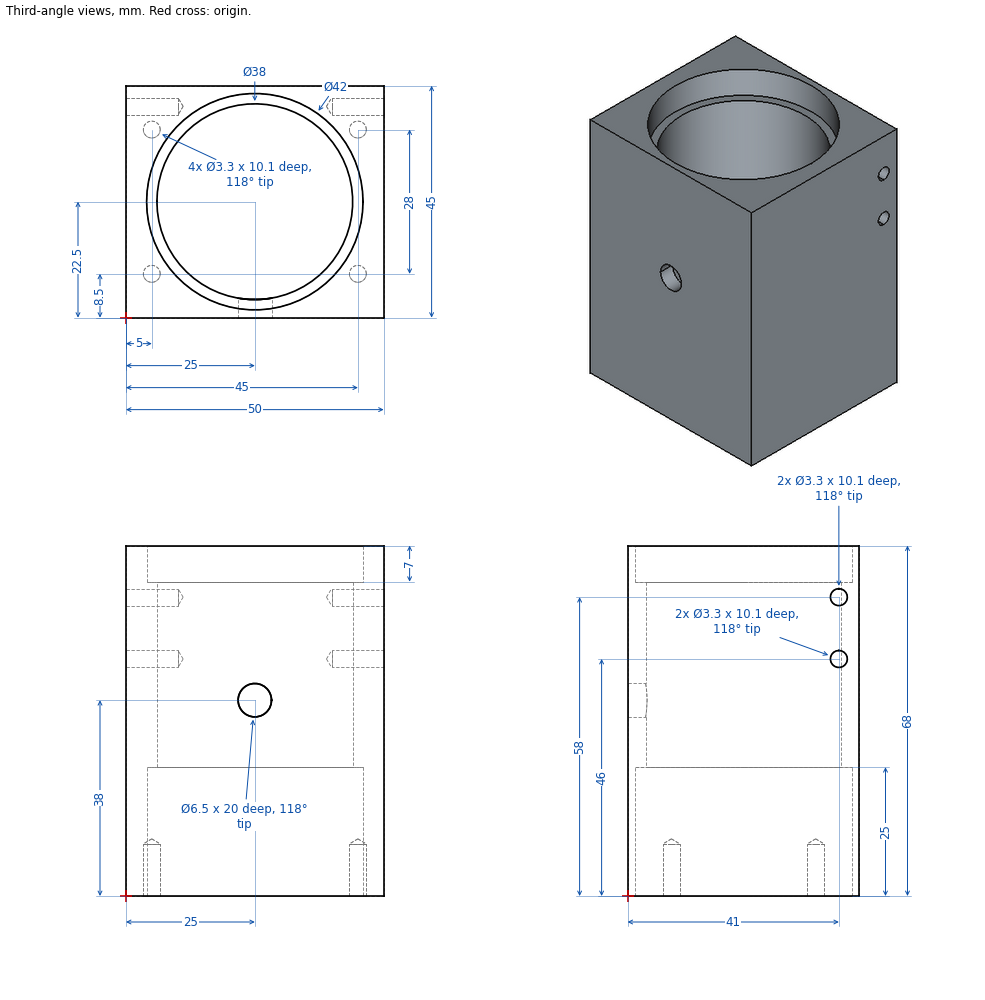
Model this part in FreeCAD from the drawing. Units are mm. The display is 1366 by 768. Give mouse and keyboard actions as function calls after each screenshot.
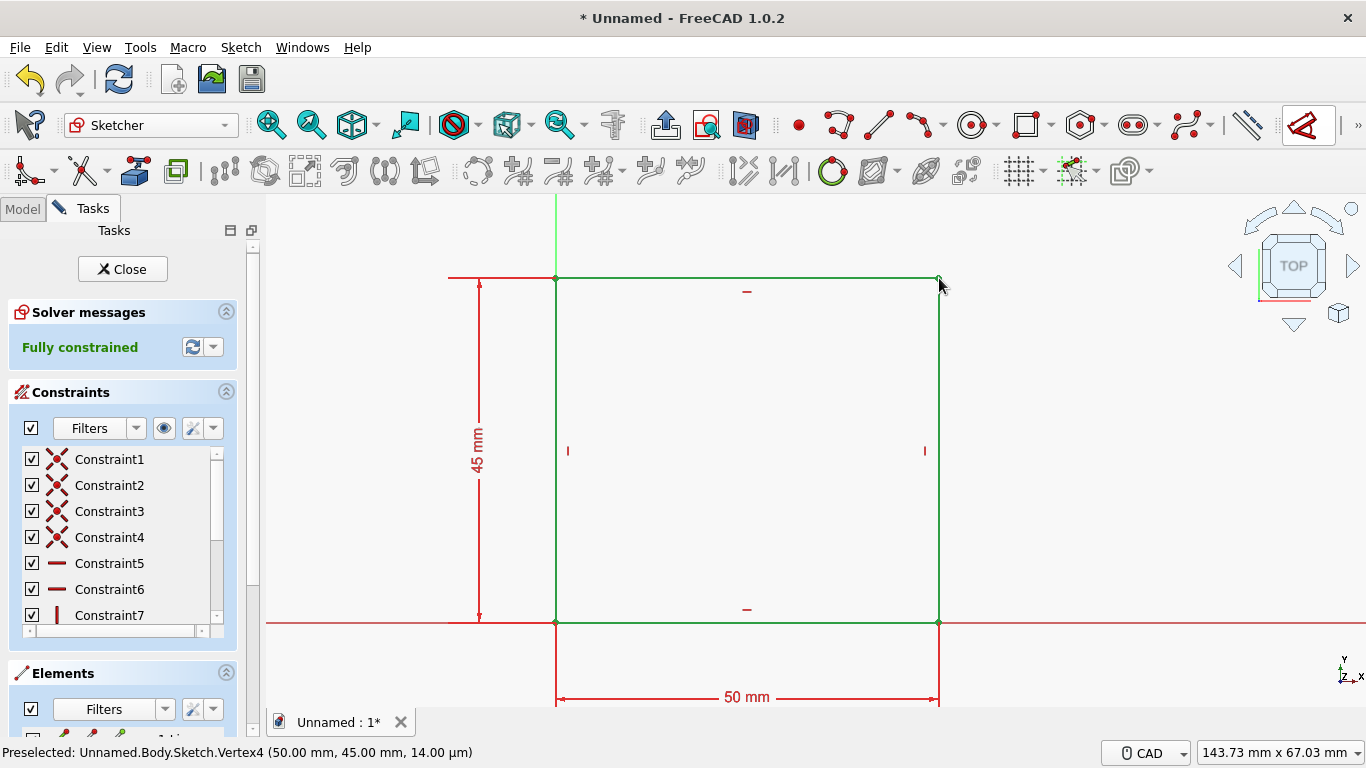
click(123, 269)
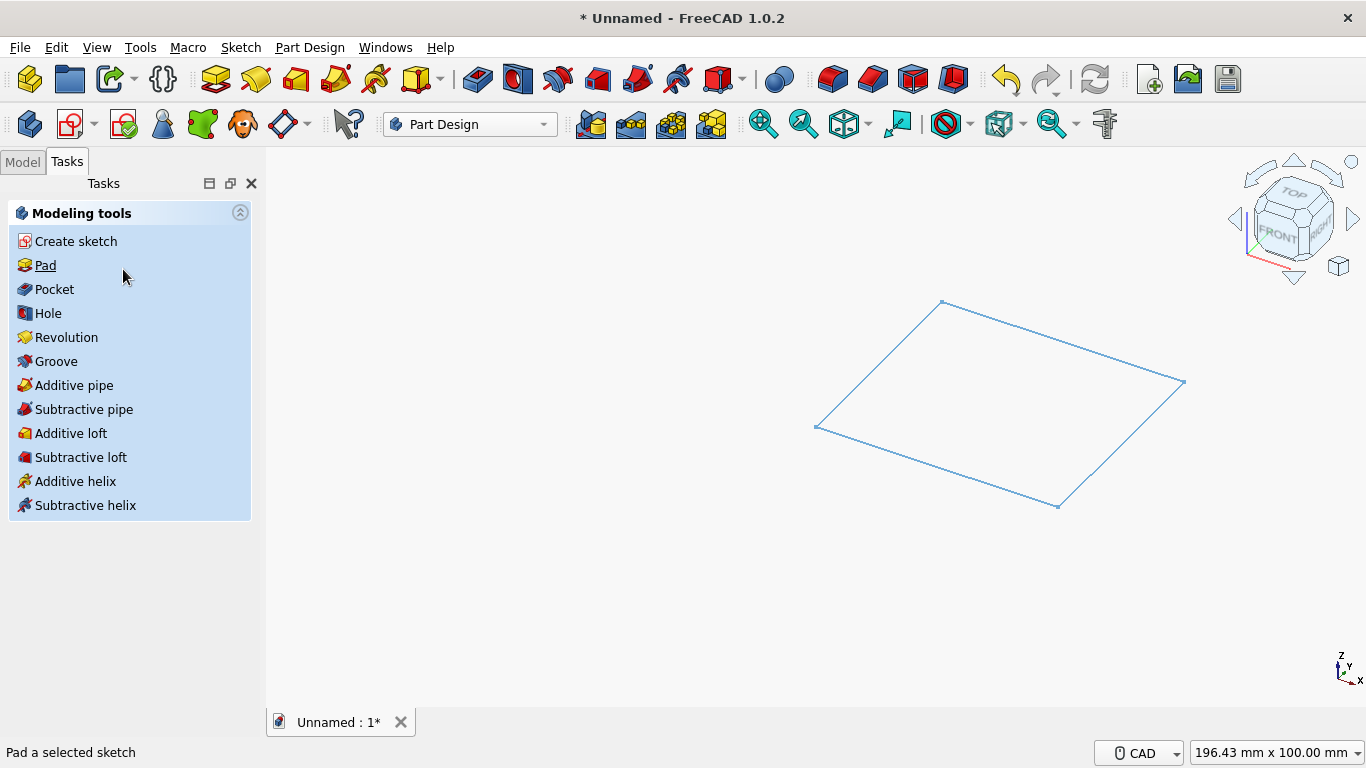
click(216, 80)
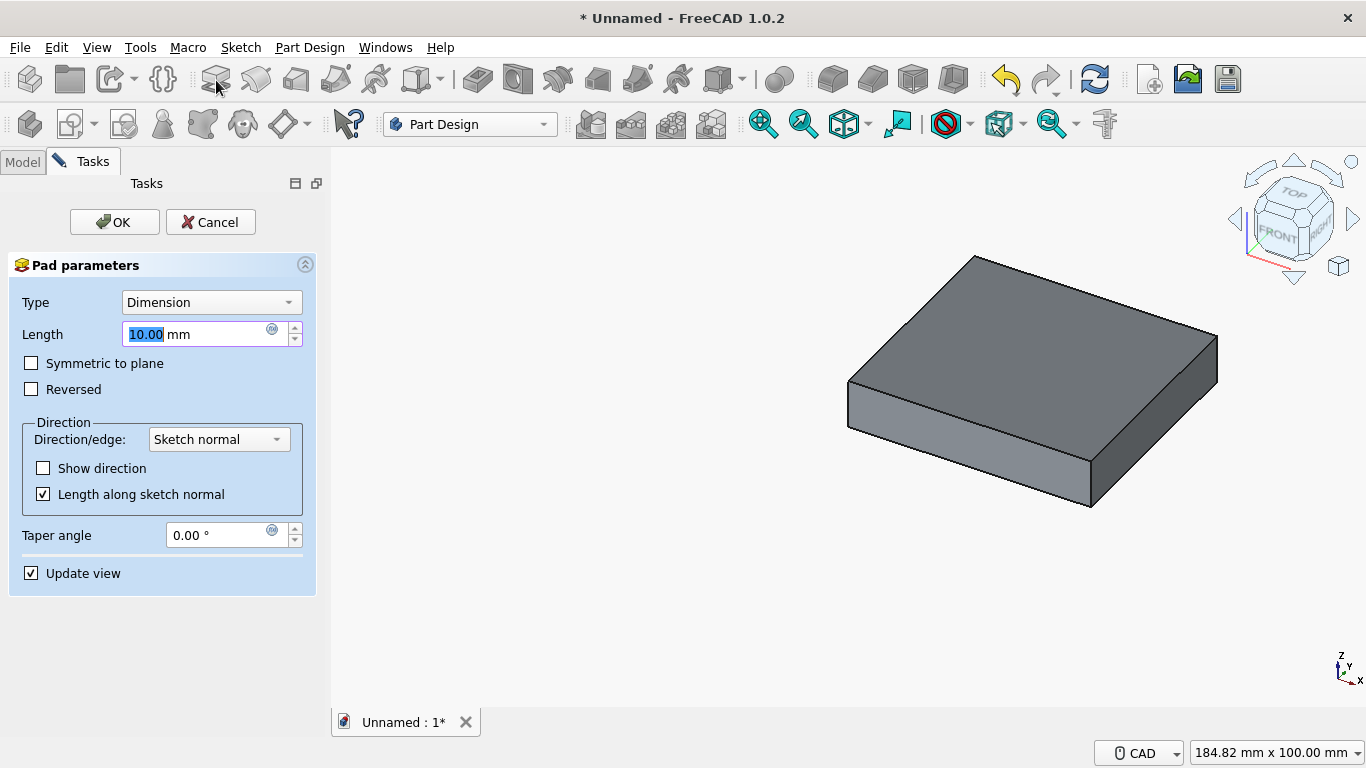
text(68)
key(Tab)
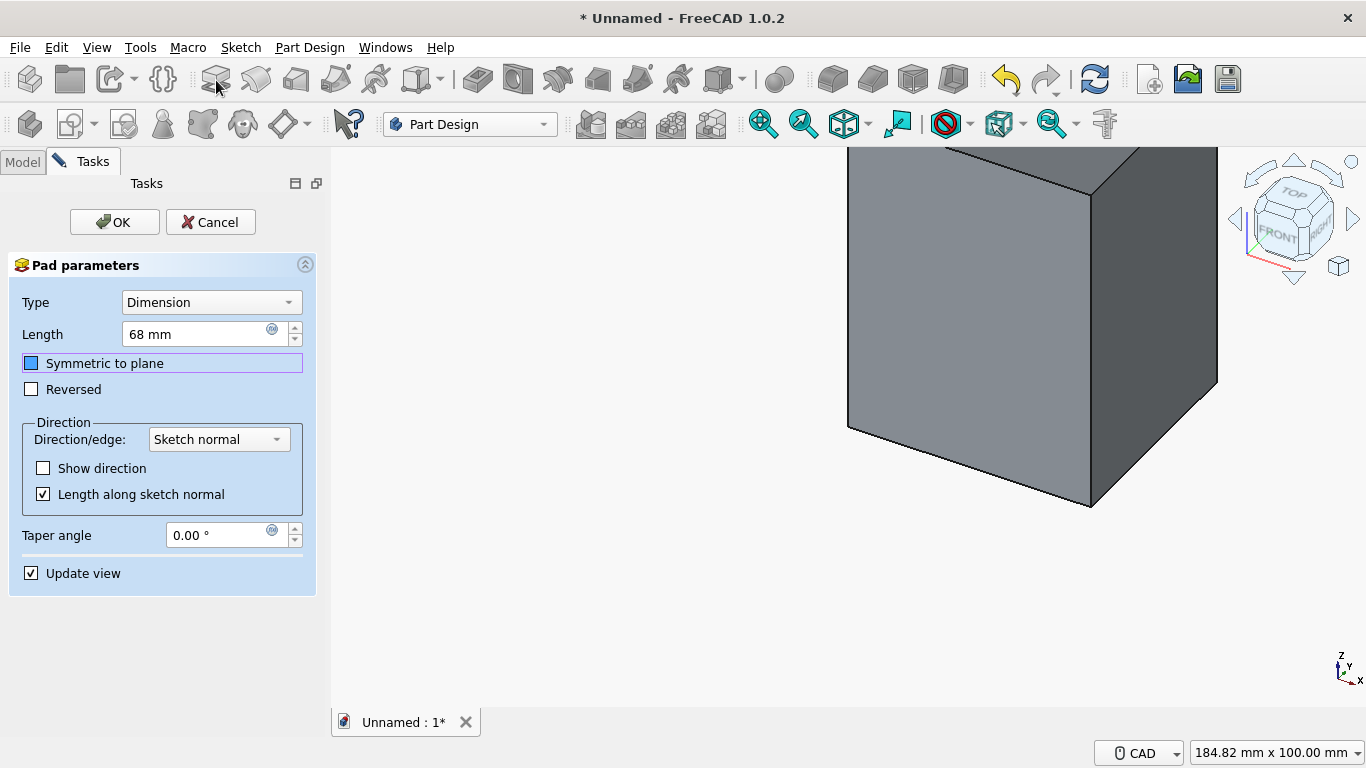
click(115, 222)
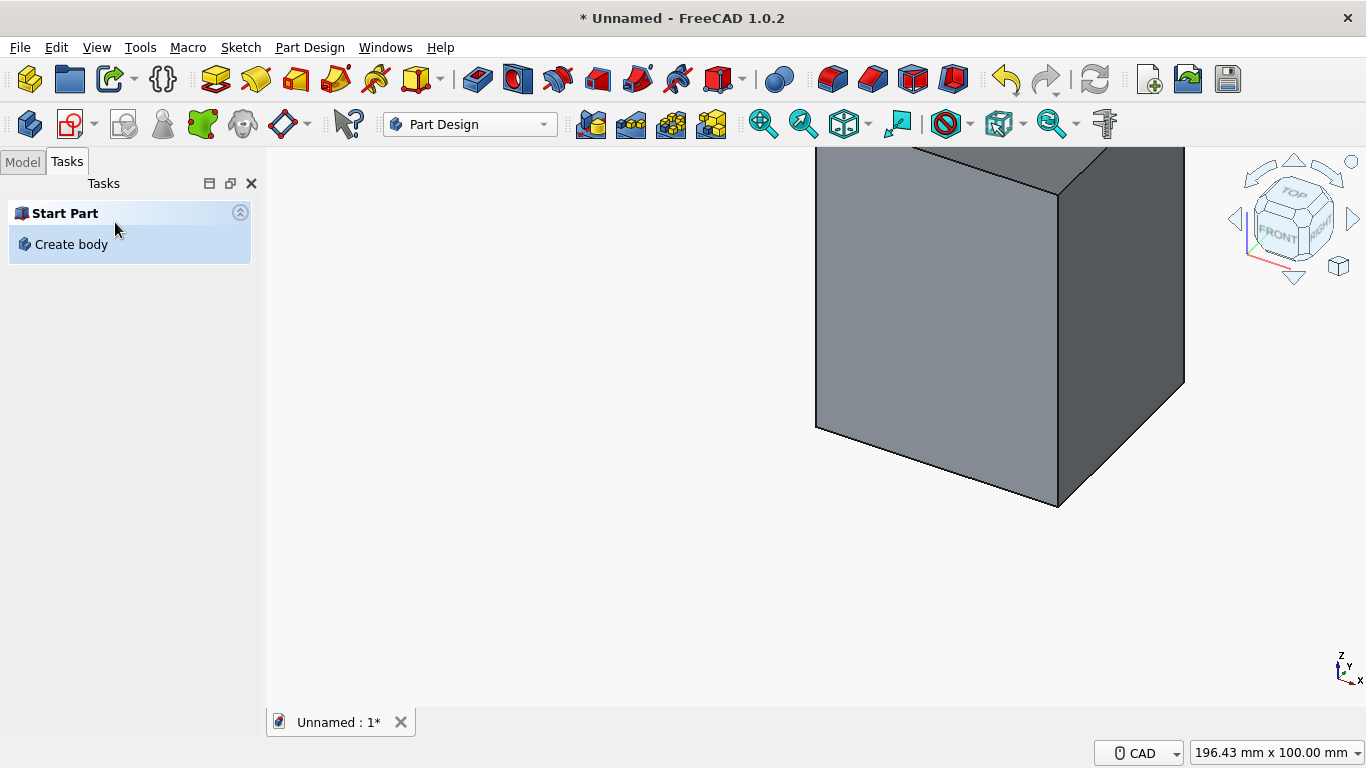
click(764, 124)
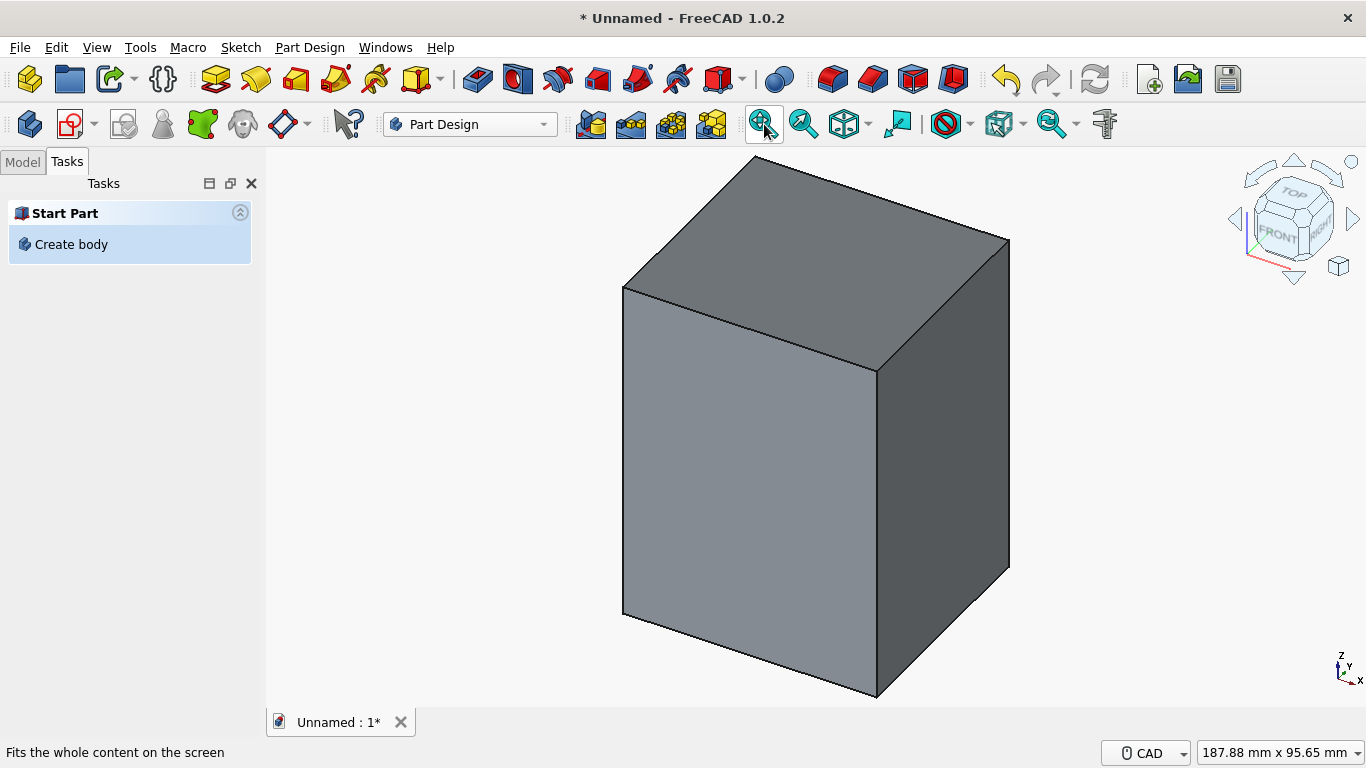
click(70, 124)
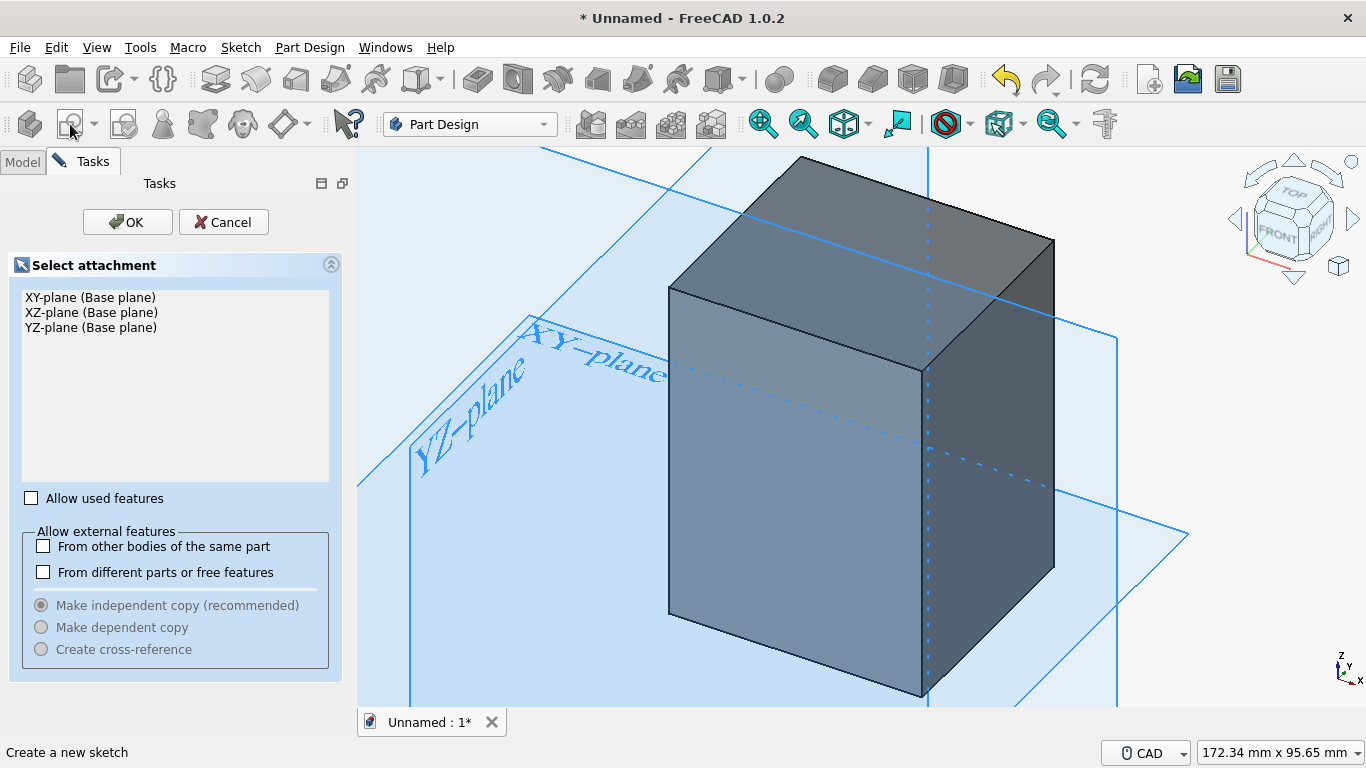
click(82, 298)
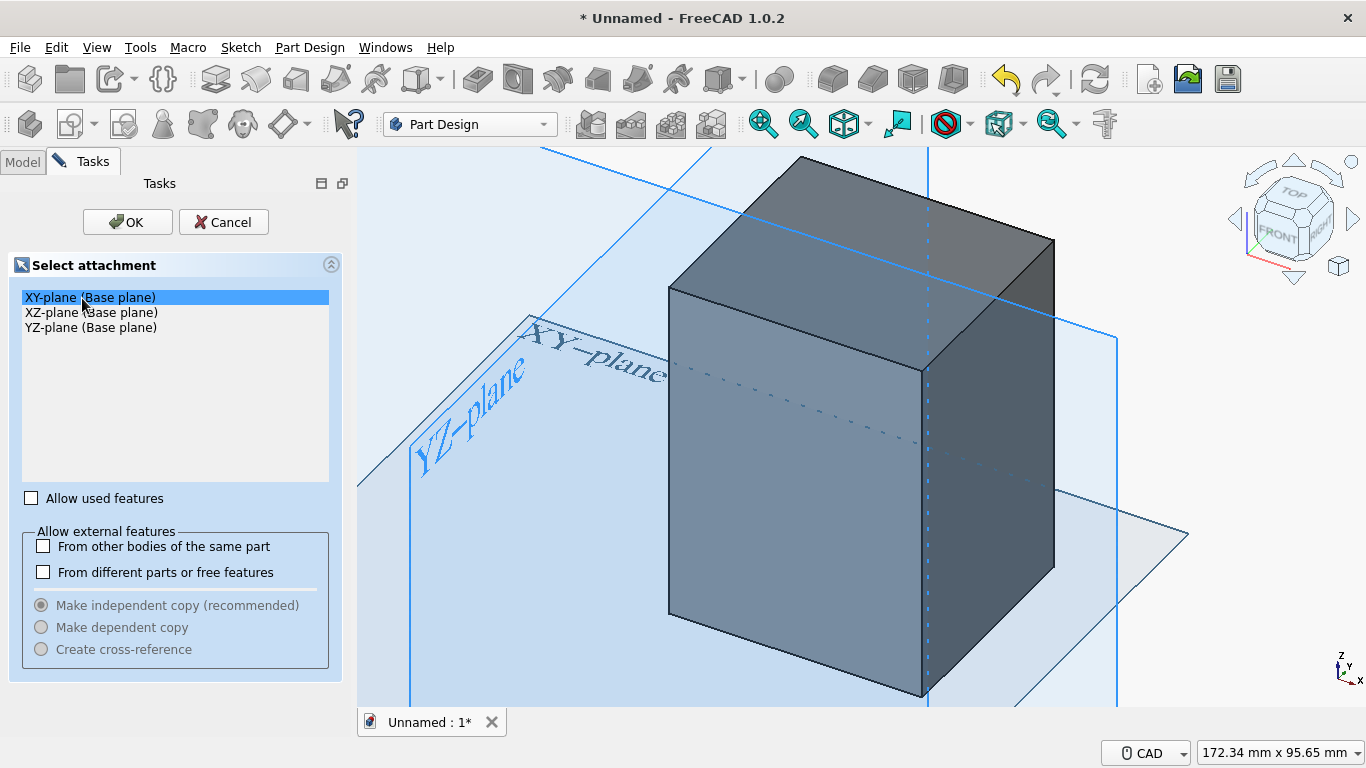
click(128, 222)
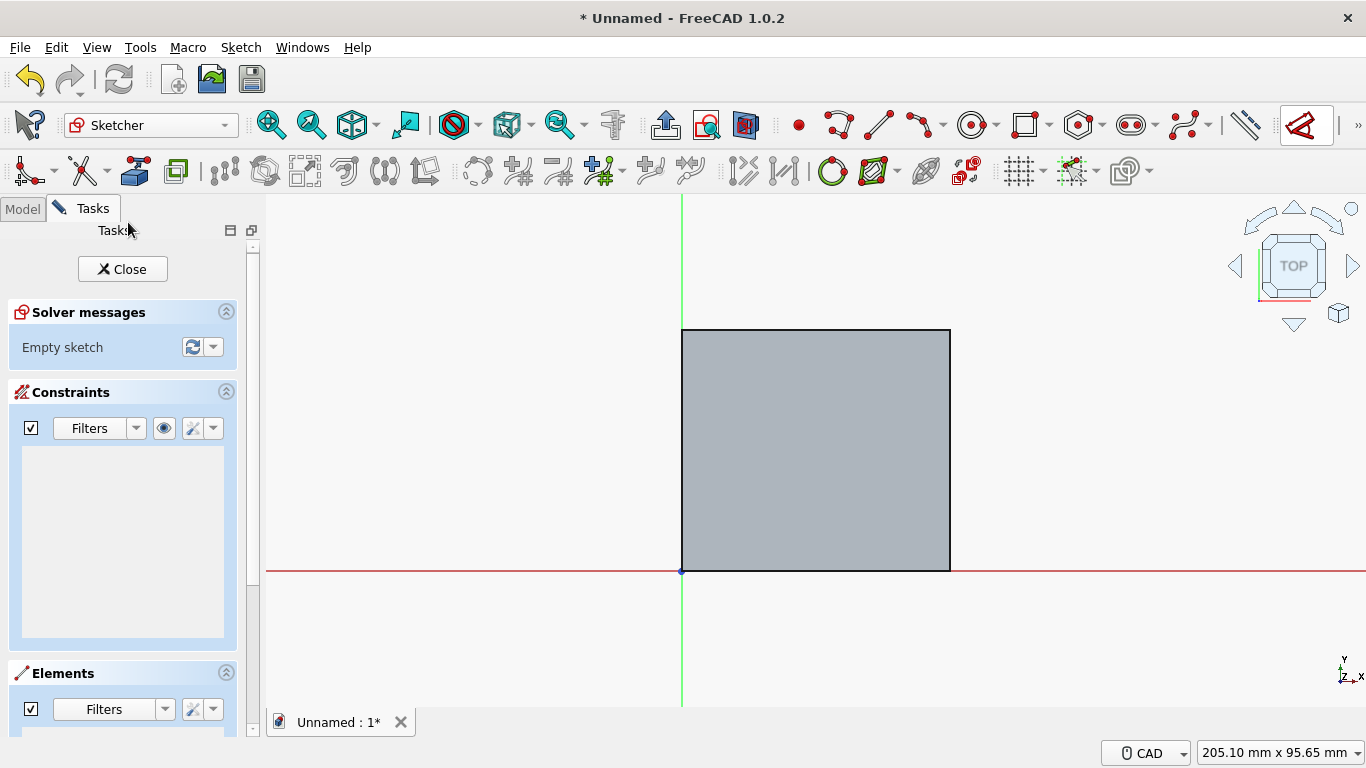
click(746, 126)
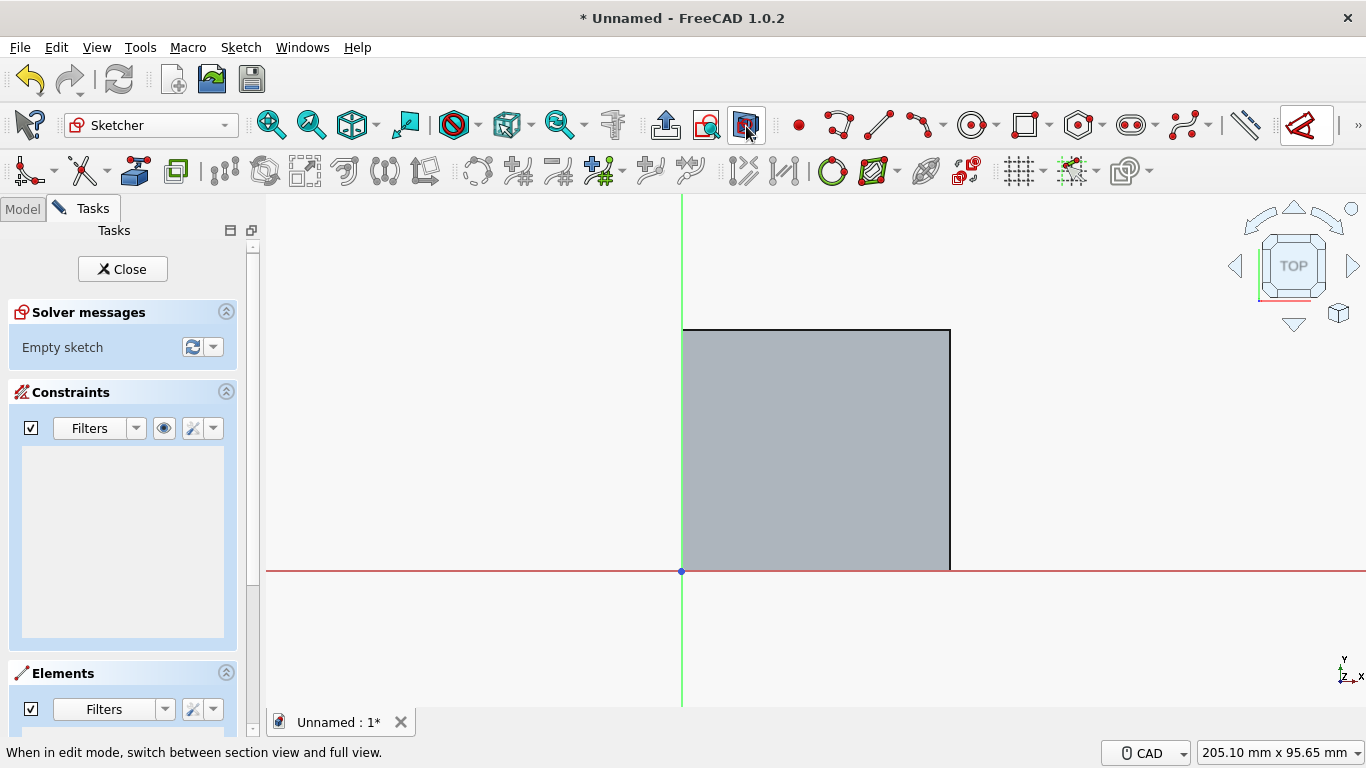
scroll(906, 479, up, 2)